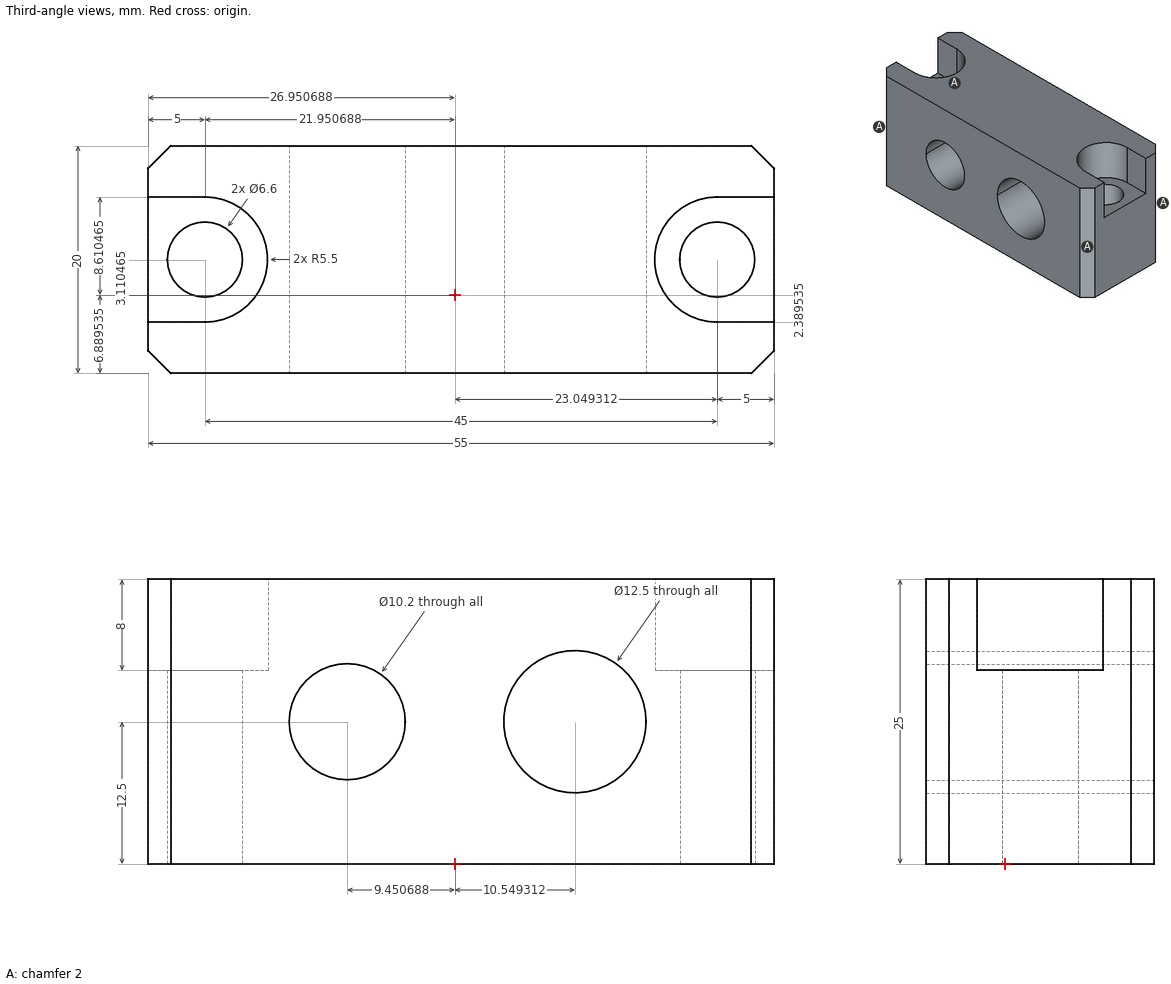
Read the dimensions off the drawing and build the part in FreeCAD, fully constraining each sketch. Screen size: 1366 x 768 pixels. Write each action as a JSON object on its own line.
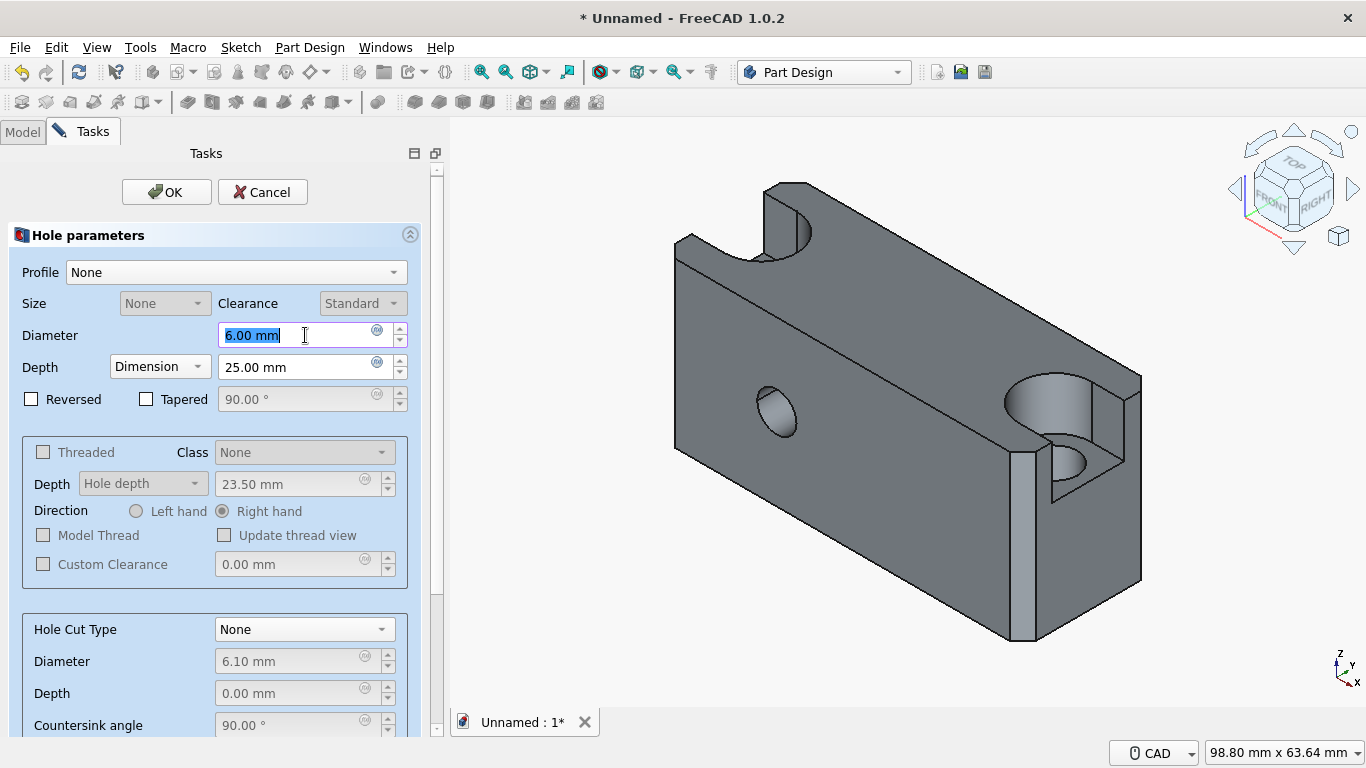
{"action": "type", "text": "10.2"}
{"action": "key", "text": "Tab"}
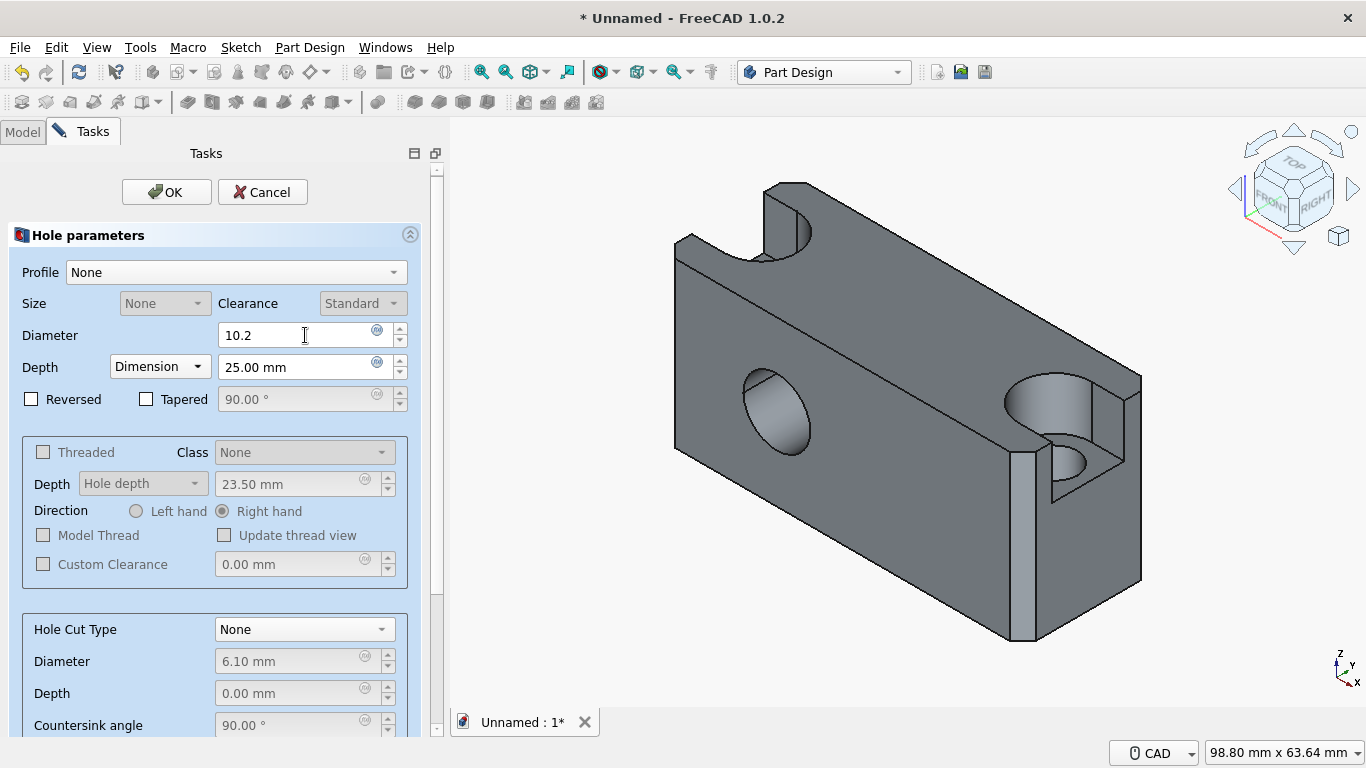
{"action": "left_click", "coordinate": [161, 366]}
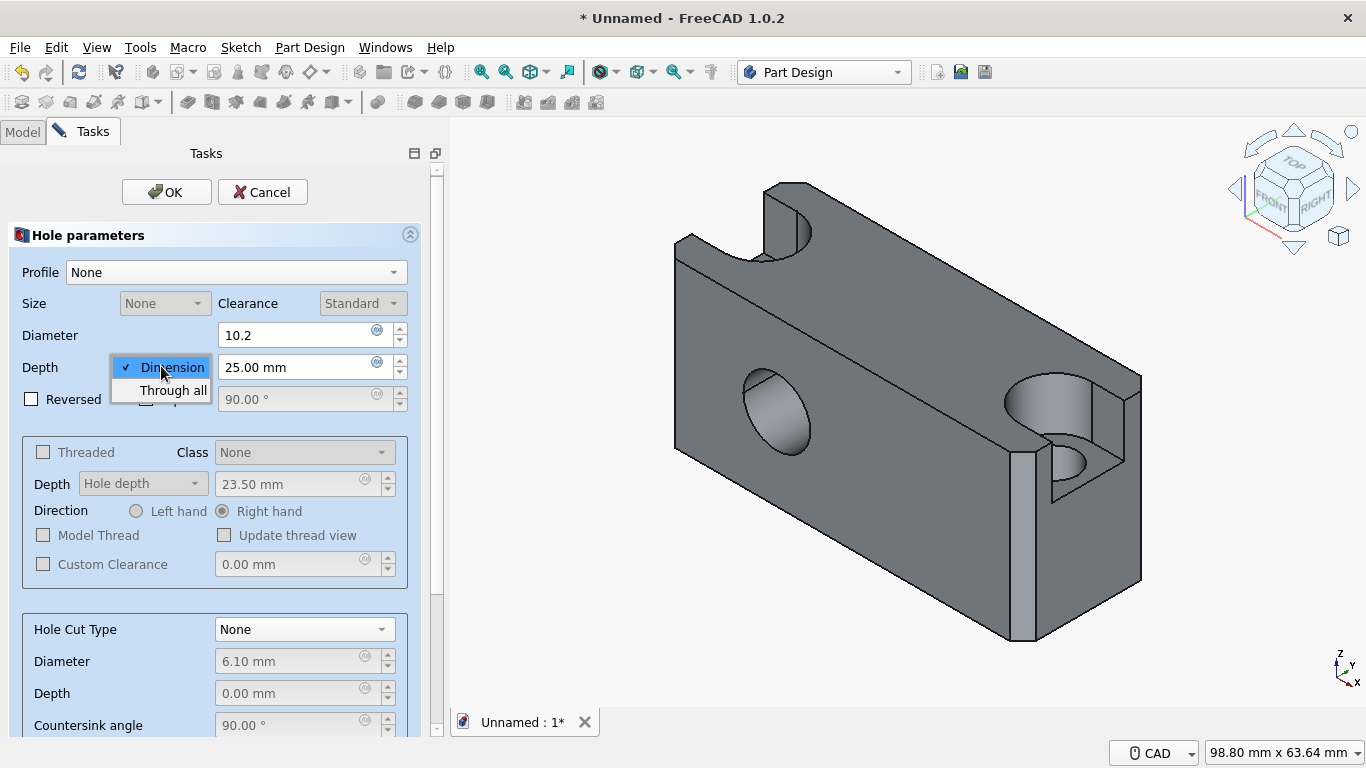
{"action": "left_click", "coordinate": [160, 390]}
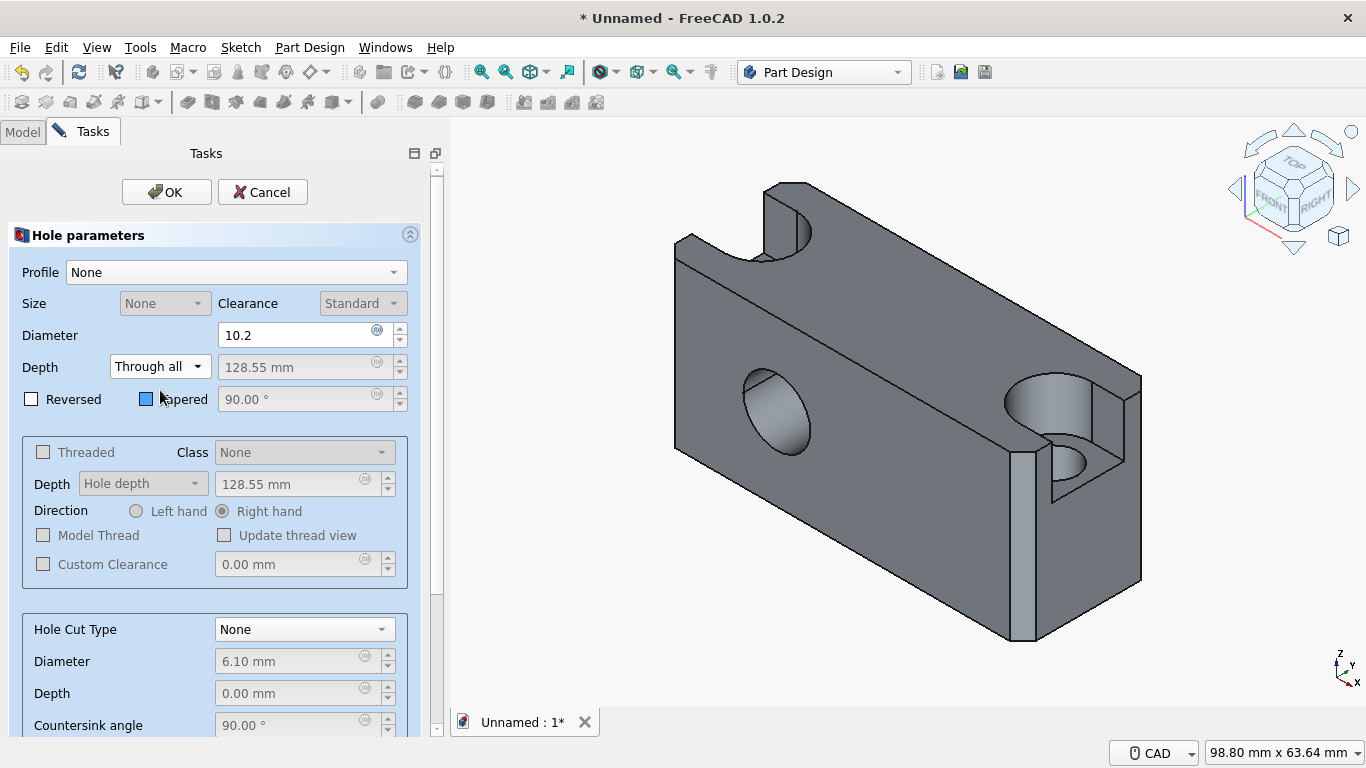
{"action": "left_click", "coordinate": [167, 192]}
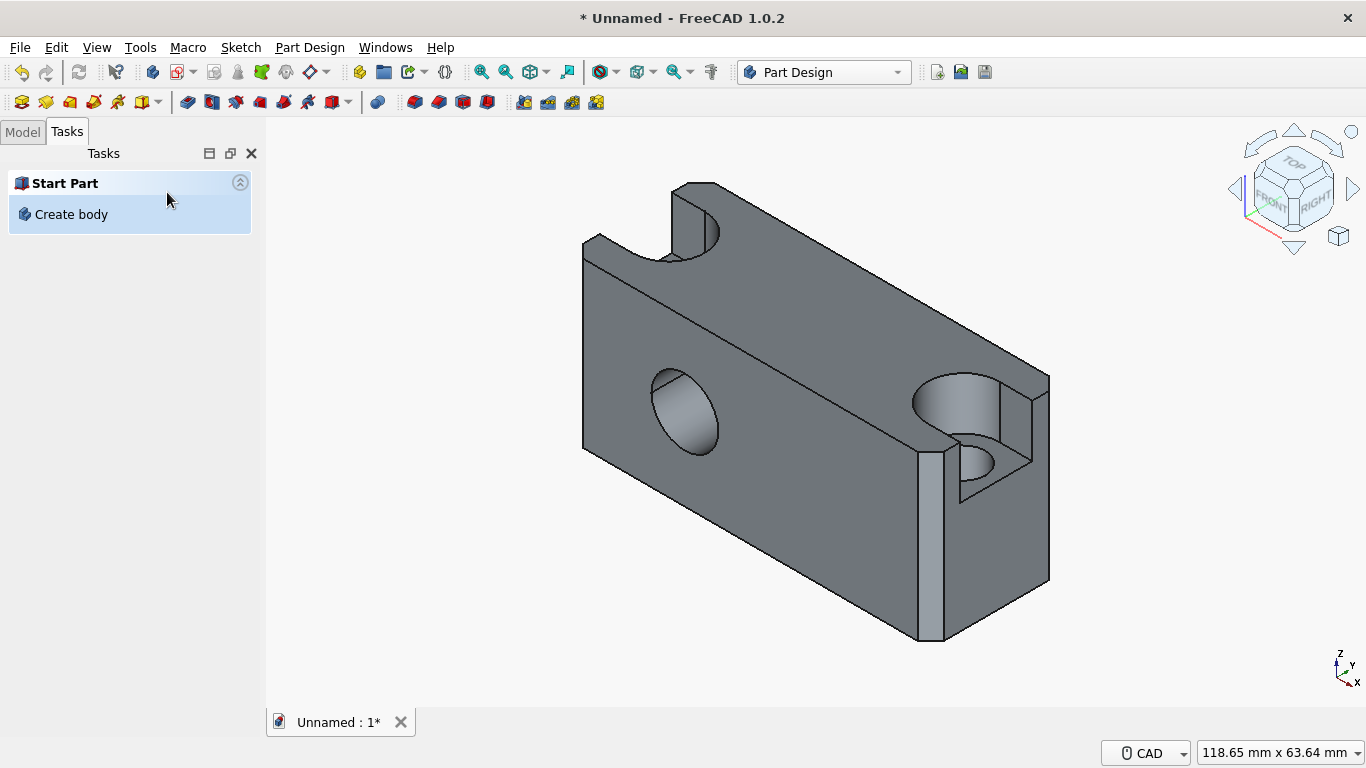
{"action": "left_click", "coordinate": [798, 476]}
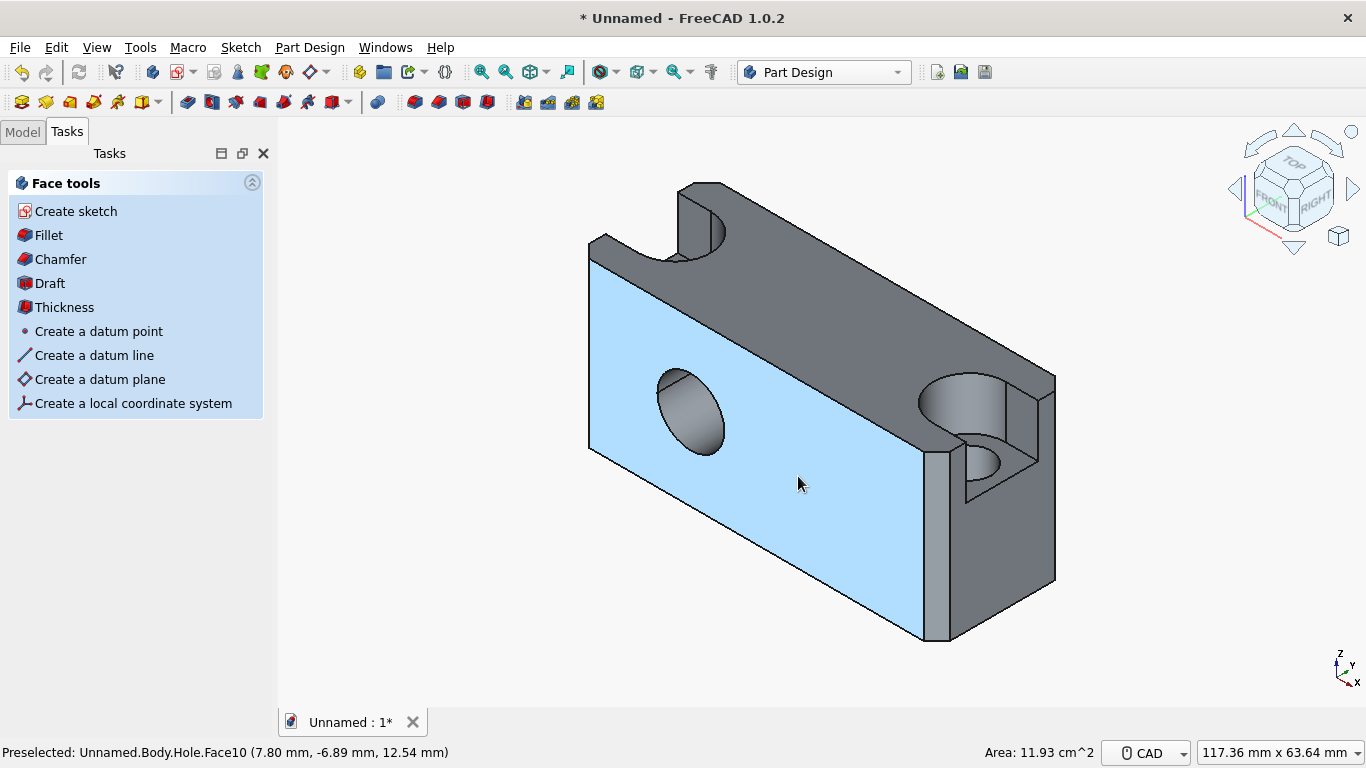
{"action": "left_click", "coordinate": [178, 72]}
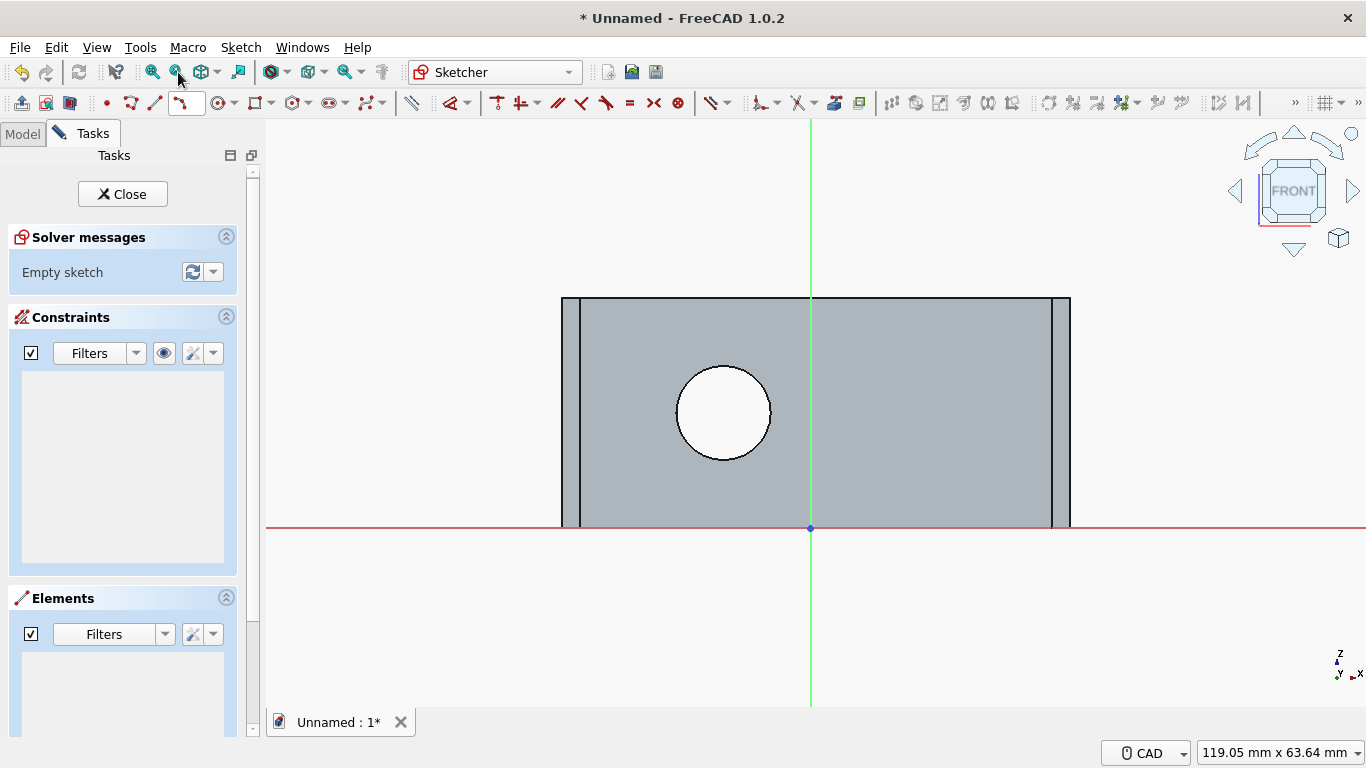
{"action": "scroll", "coordinate": [1004, 465], "scroll_direction": "up", "scroll_amount": 4}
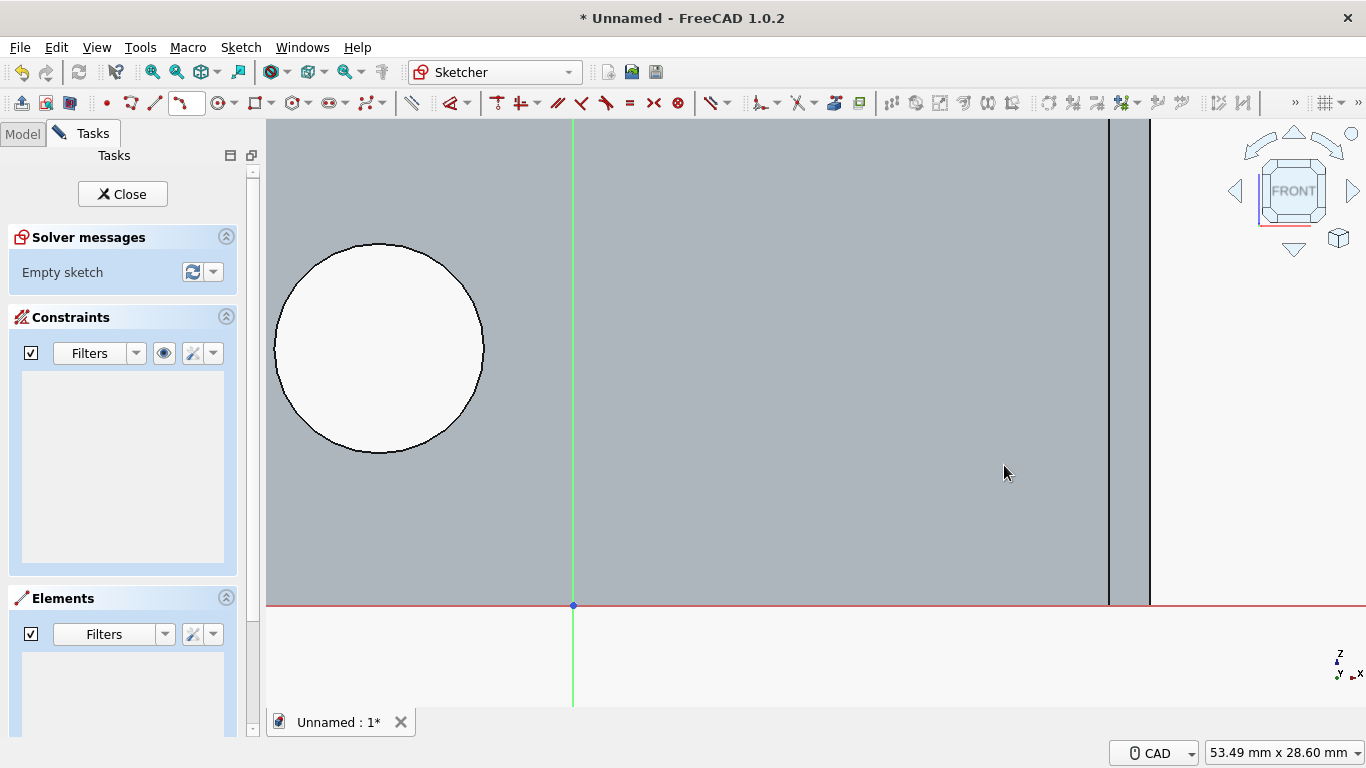
{"action": "key", "text": "g c"}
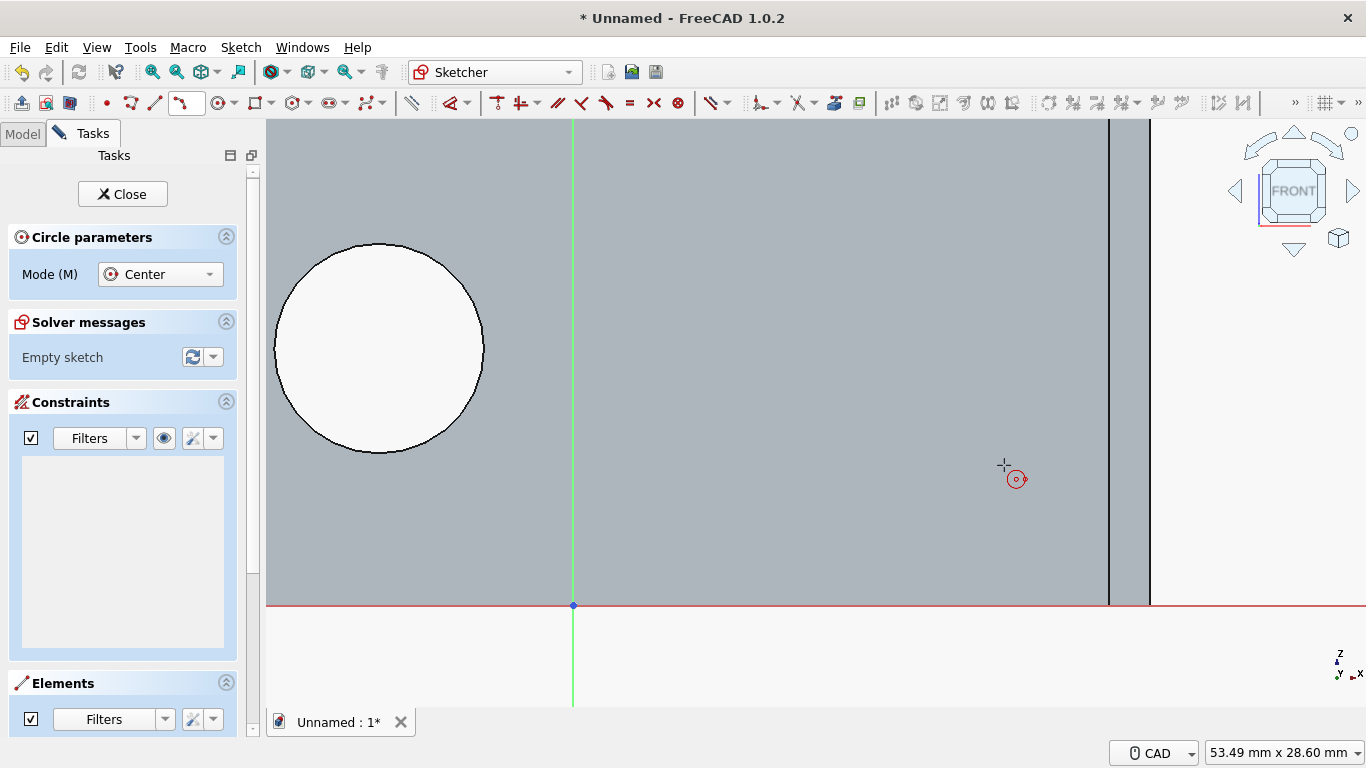
{"action": "left_click", "coordinate": [790, 349]}
{"action": "left_click", "coordinate": [881, 258]}
{"action": "key", "text": "Escape"}